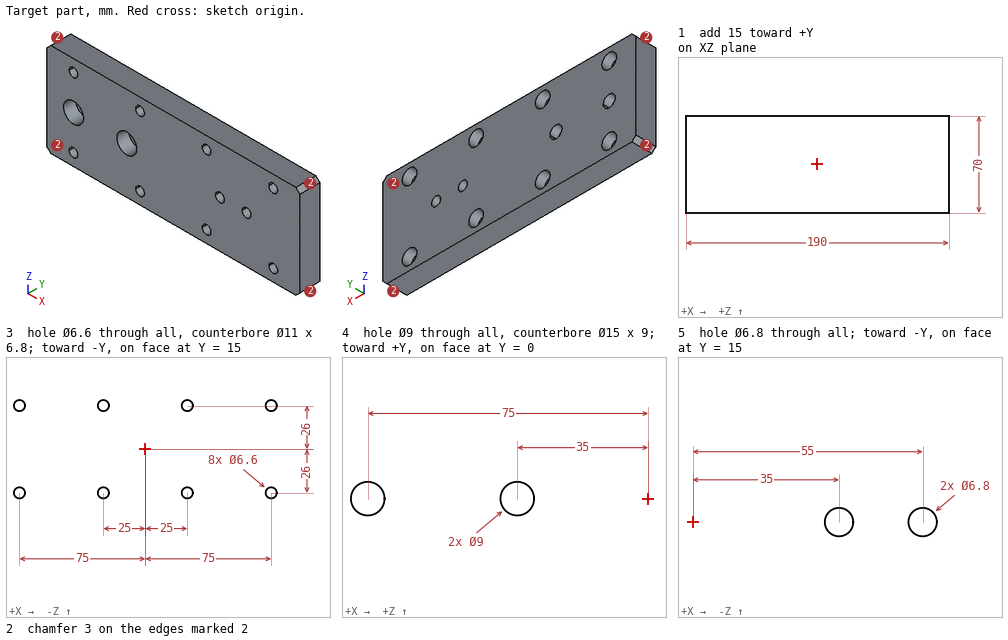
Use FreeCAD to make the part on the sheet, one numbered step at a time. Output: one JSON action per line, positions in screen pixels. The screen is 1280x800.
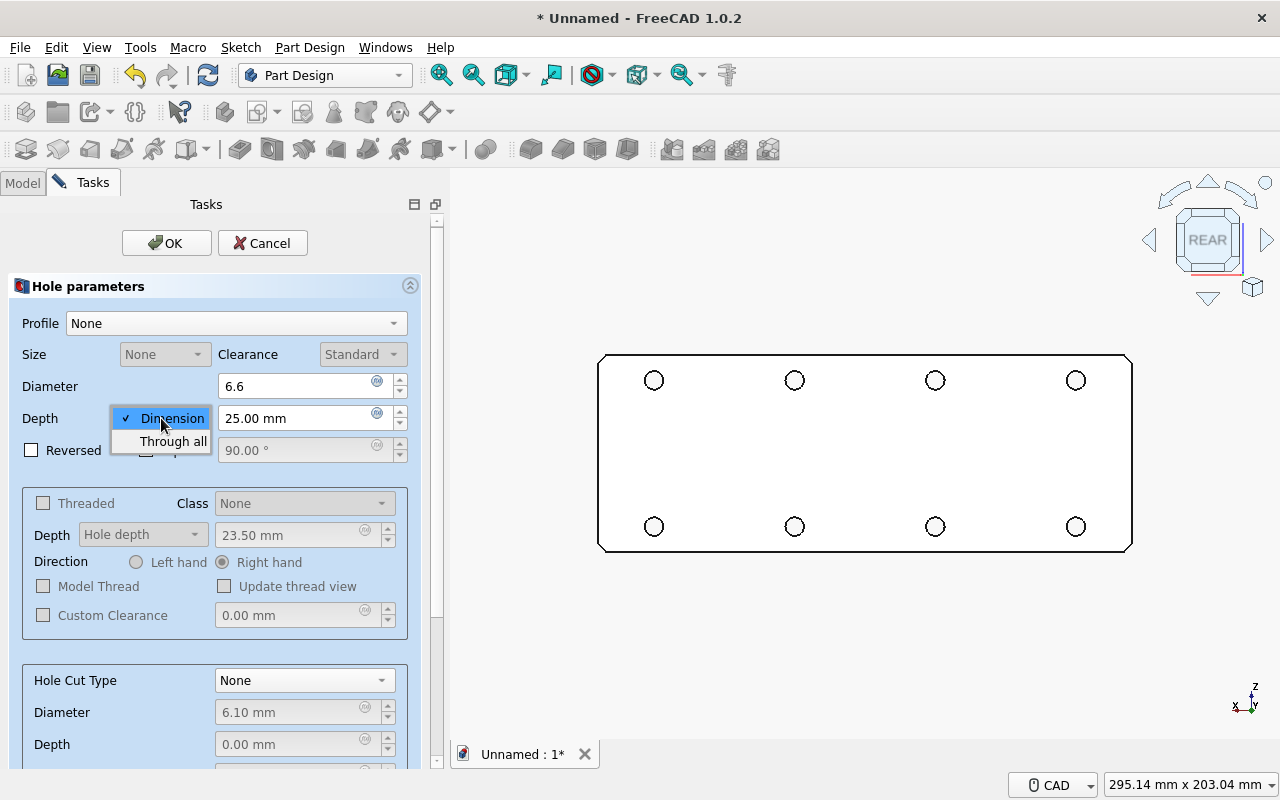
{"action": "left_click", "coordinate": [160, 442]}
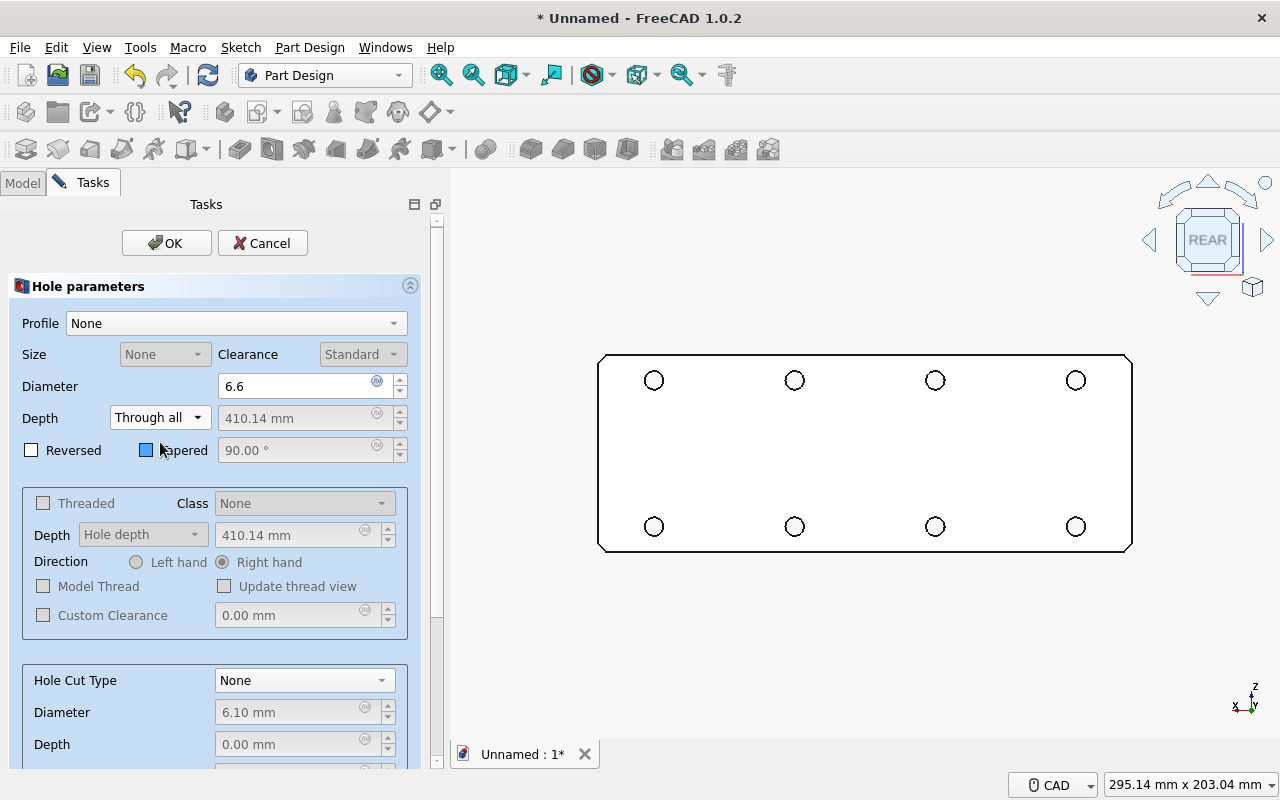
{"action": "left_click", "coordinate": [306, 680]}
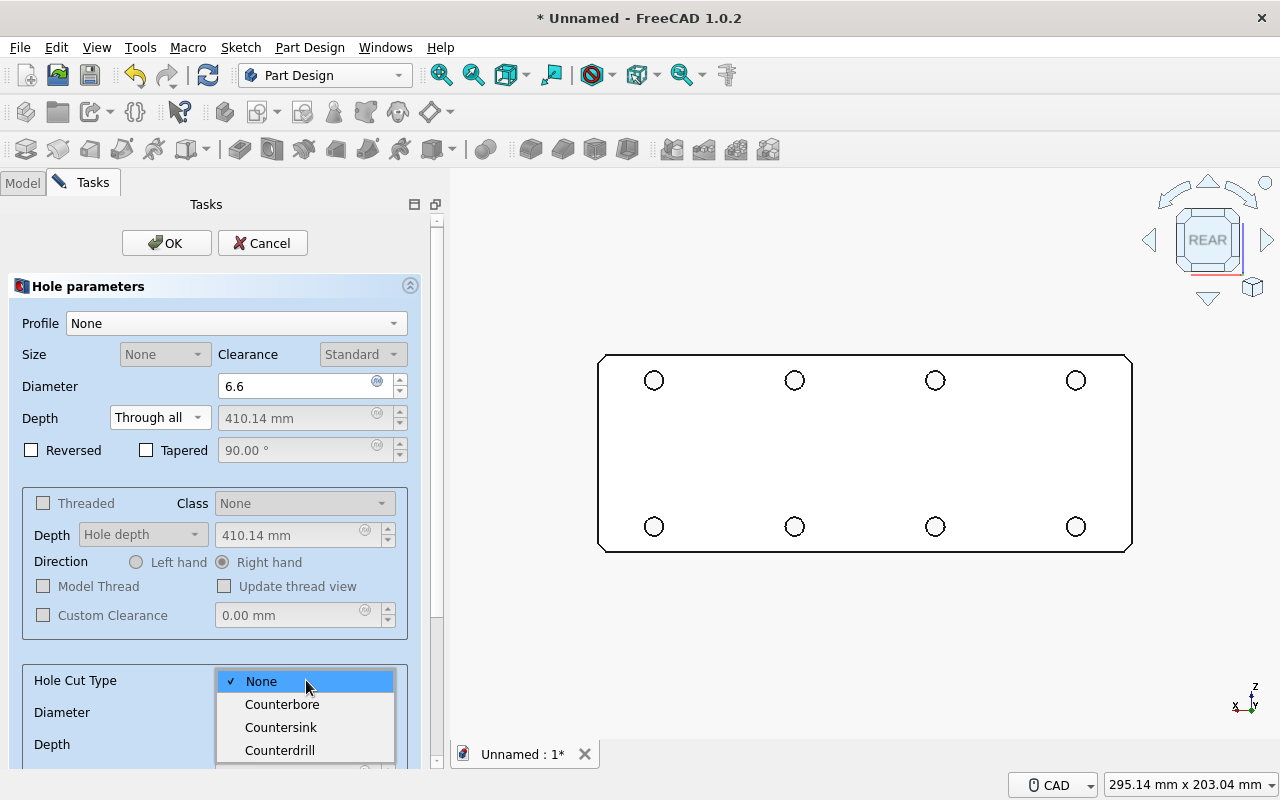
{"action": "left_click", "coordinate": [304, 704]}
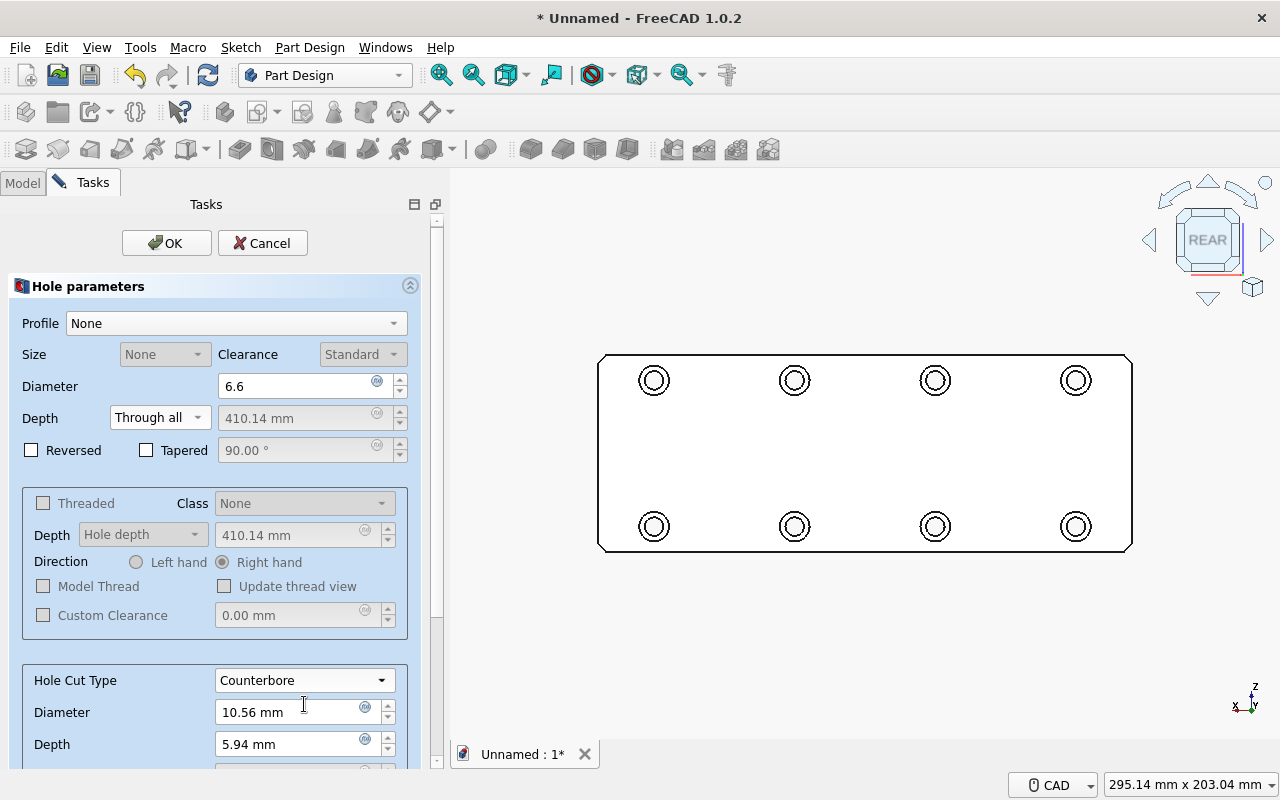
{"action": "triple_click", "coordinate": [298, 712]}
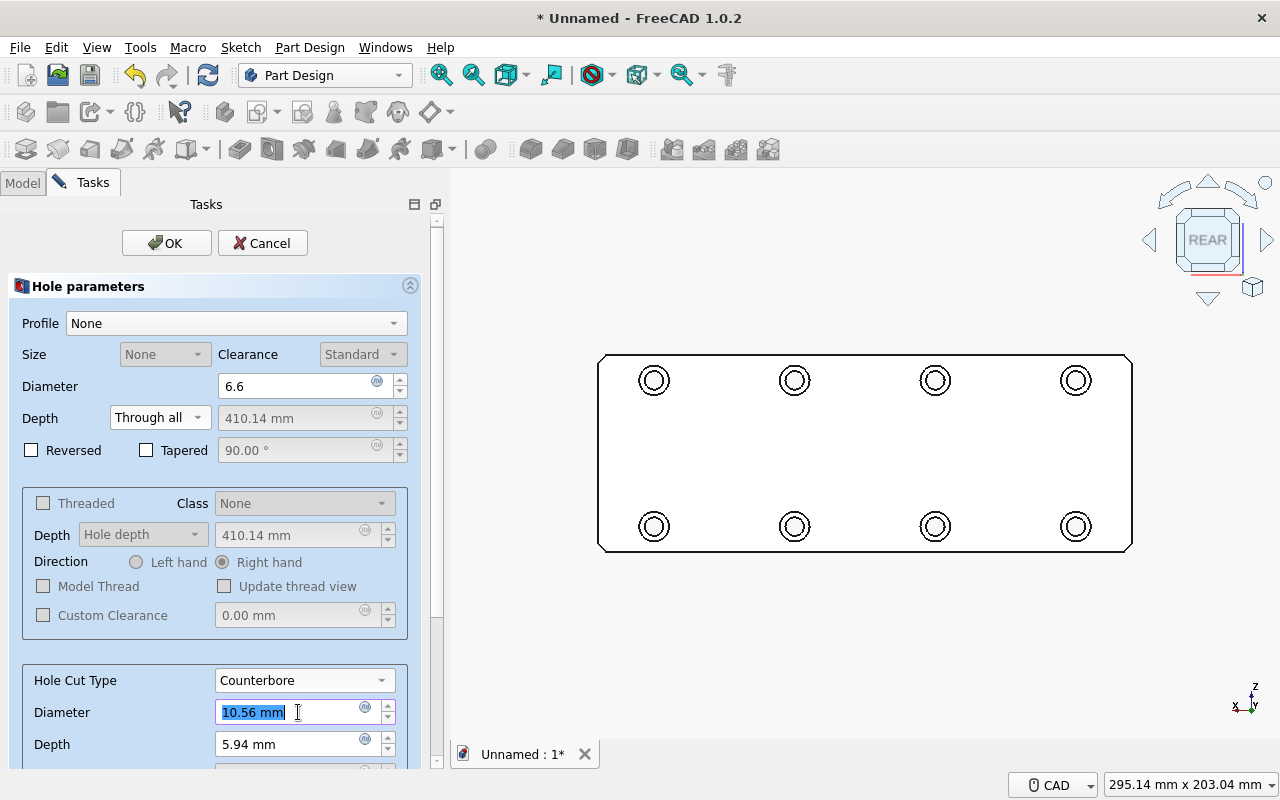
{"action": "type", "text": "11"}
{"action": "key", "text": "Tab"}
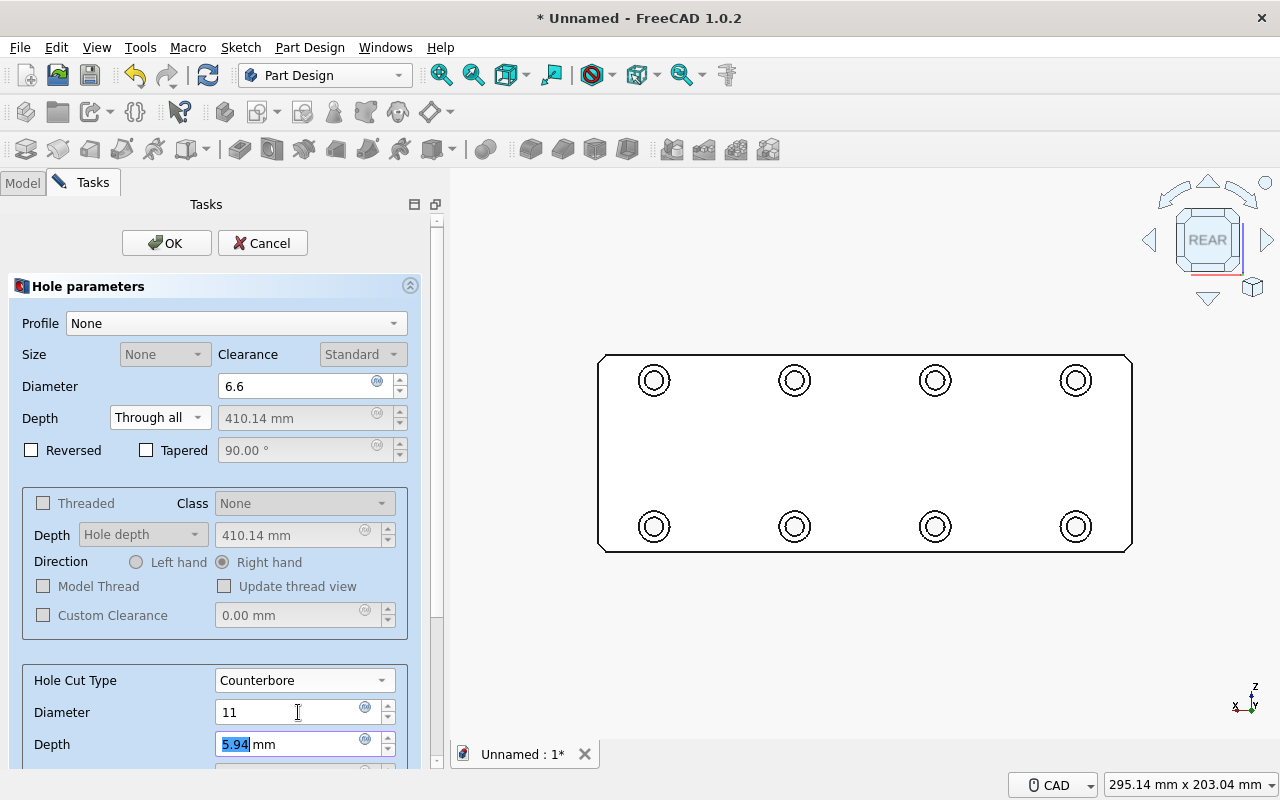
{"action": "type", "text": "6.8"}
{"action": "key", "text": "Tab"}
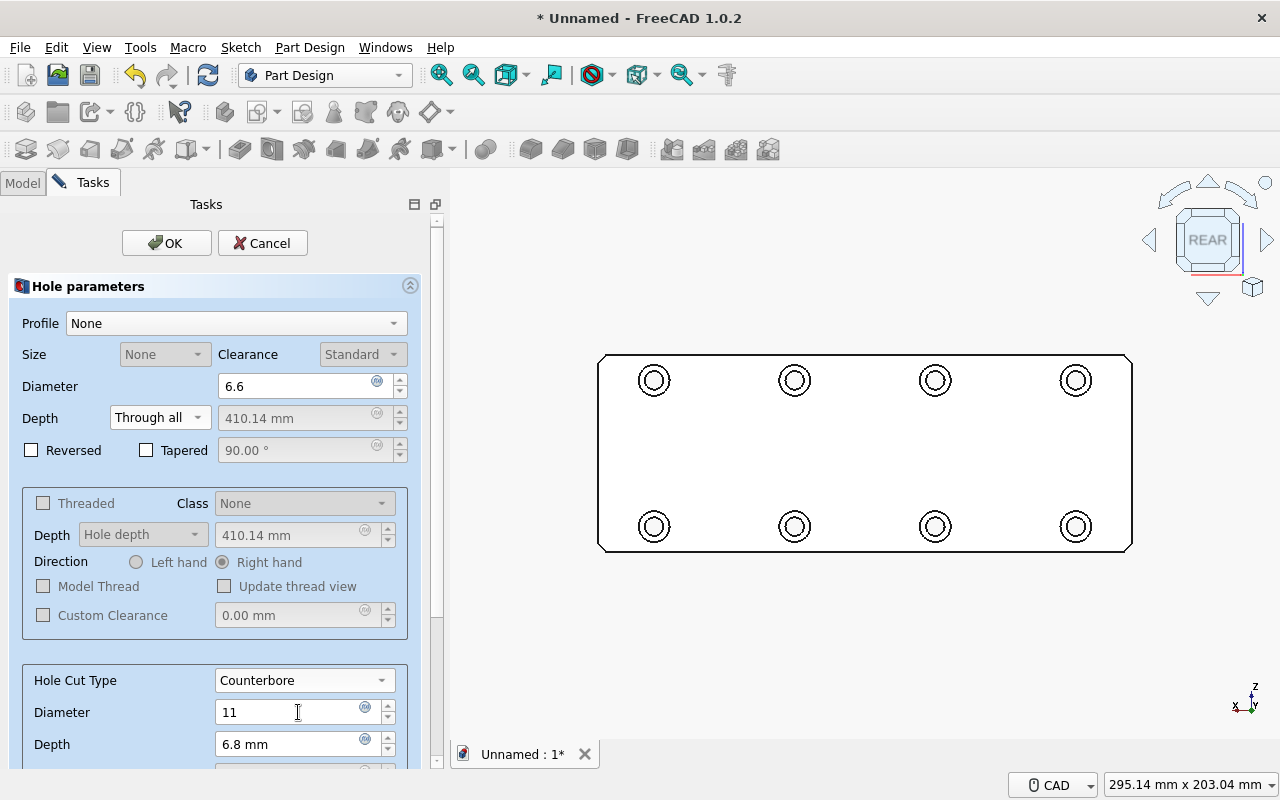
{"action": "left_click", "coordinate": [167, 243]}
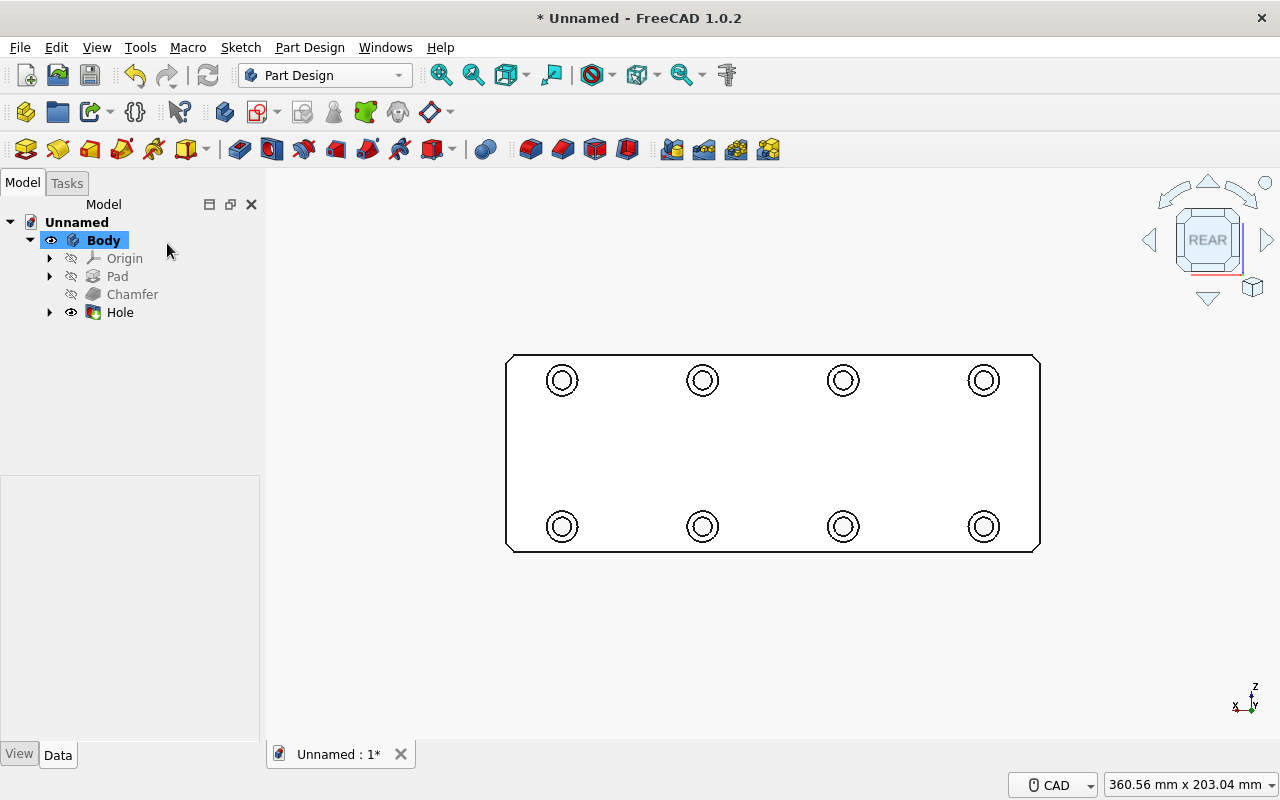
{"action": "key", "text": "0"}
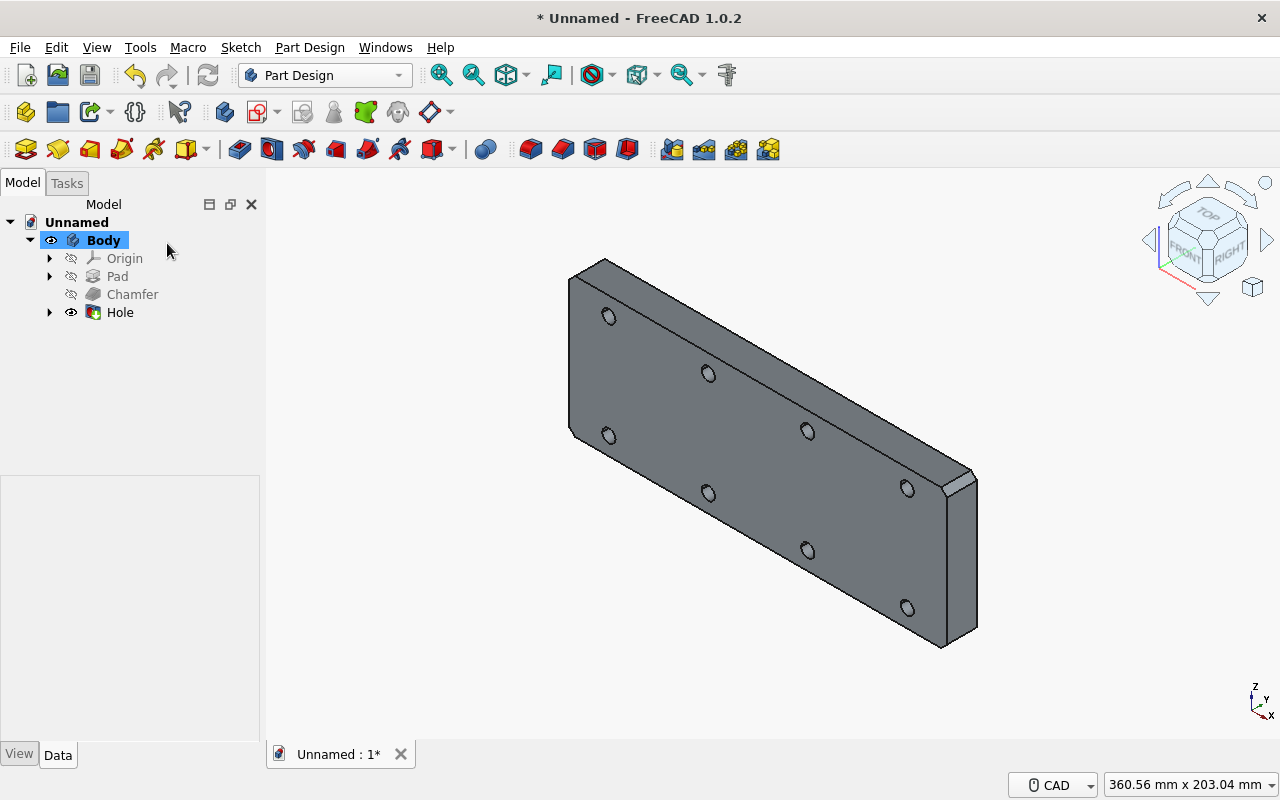
{"action": "left_click", "coordinate": [758, 461]}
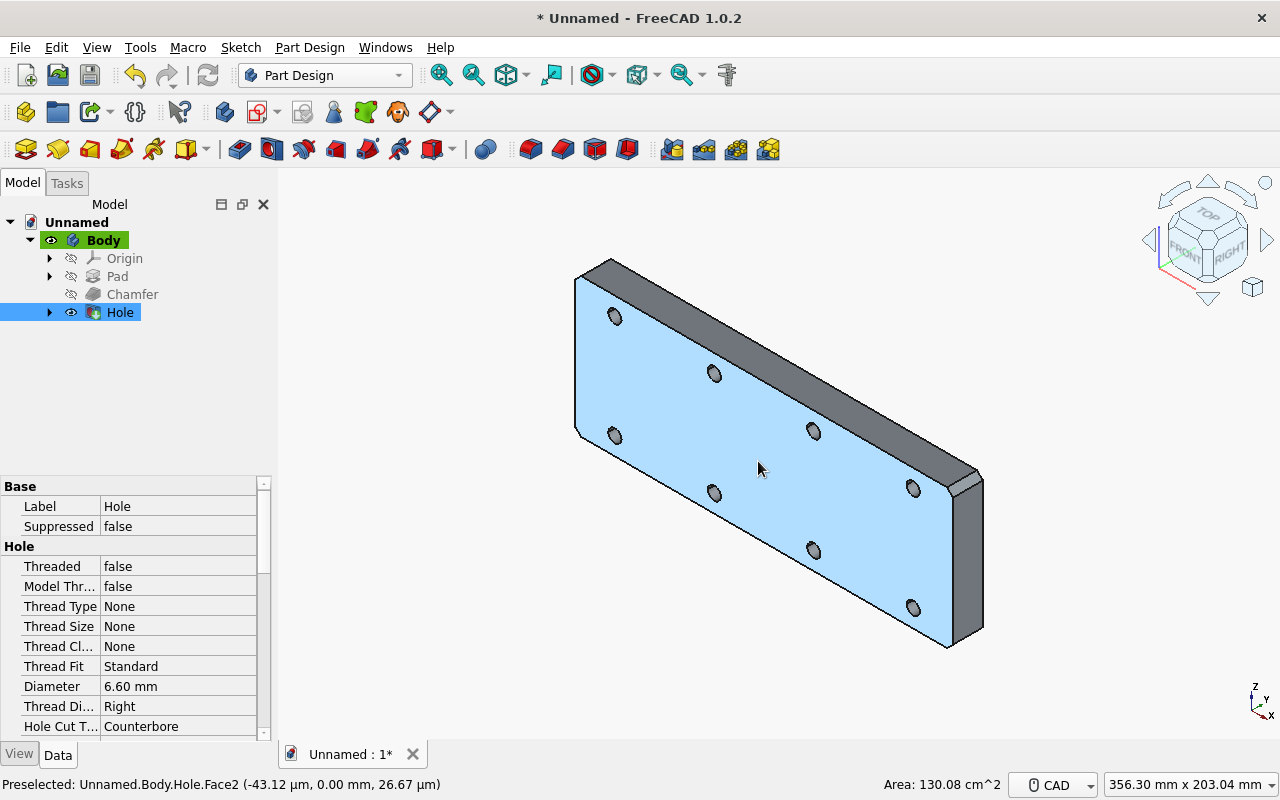
{"action": "left_click", "coordinate": [258, 112]}